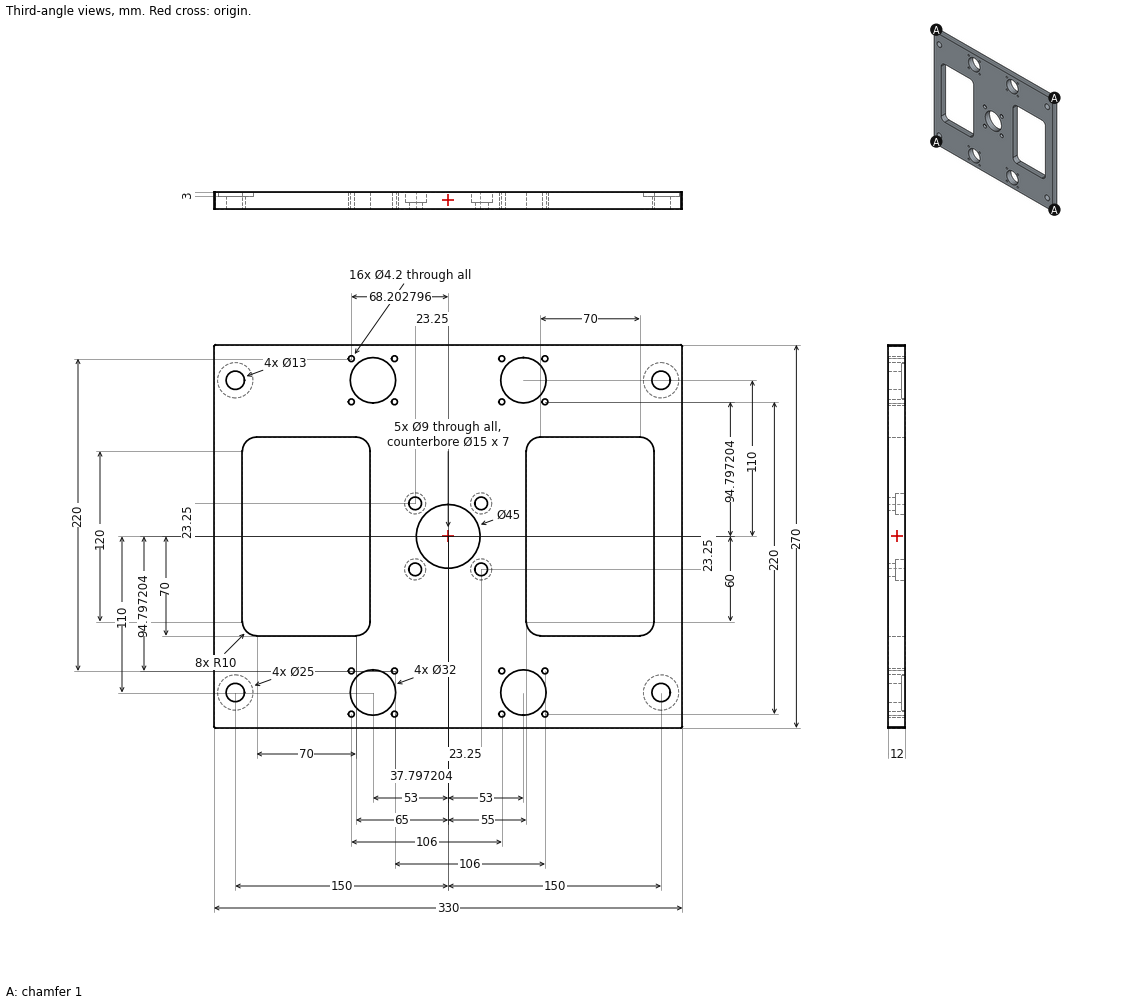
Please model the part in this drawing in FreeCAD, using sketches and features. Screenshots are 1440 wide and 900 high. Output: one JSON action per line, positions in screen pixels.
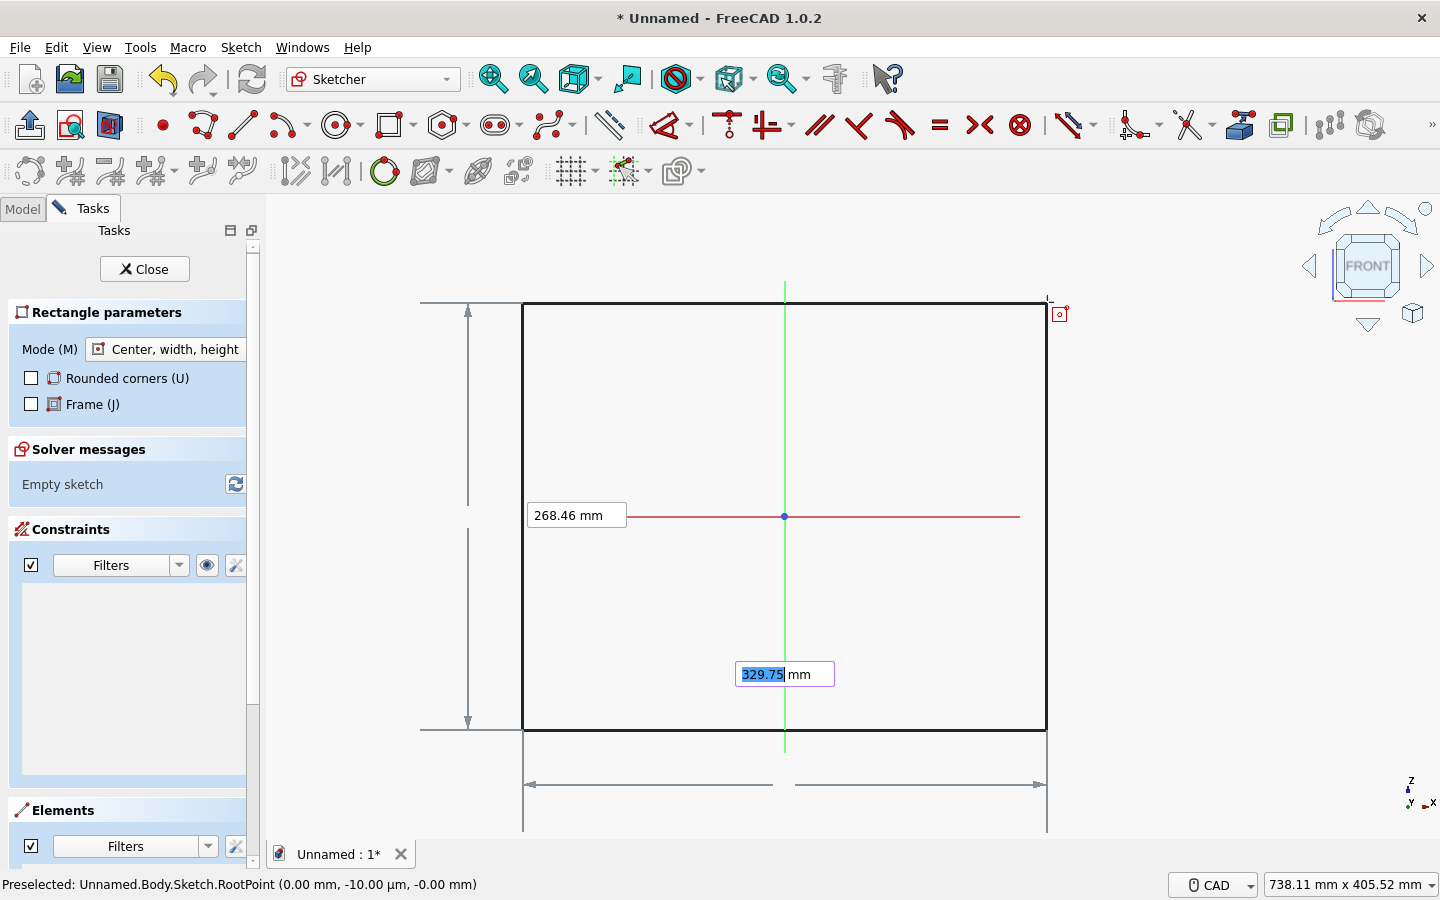
{"action": "type", "text": "330"}
{"action": "key", "text": "Tab"}
{"action": "type", "text": "270"}
{"action": "key", "text": "Return"}
{"action": "key", "text": "Escape"}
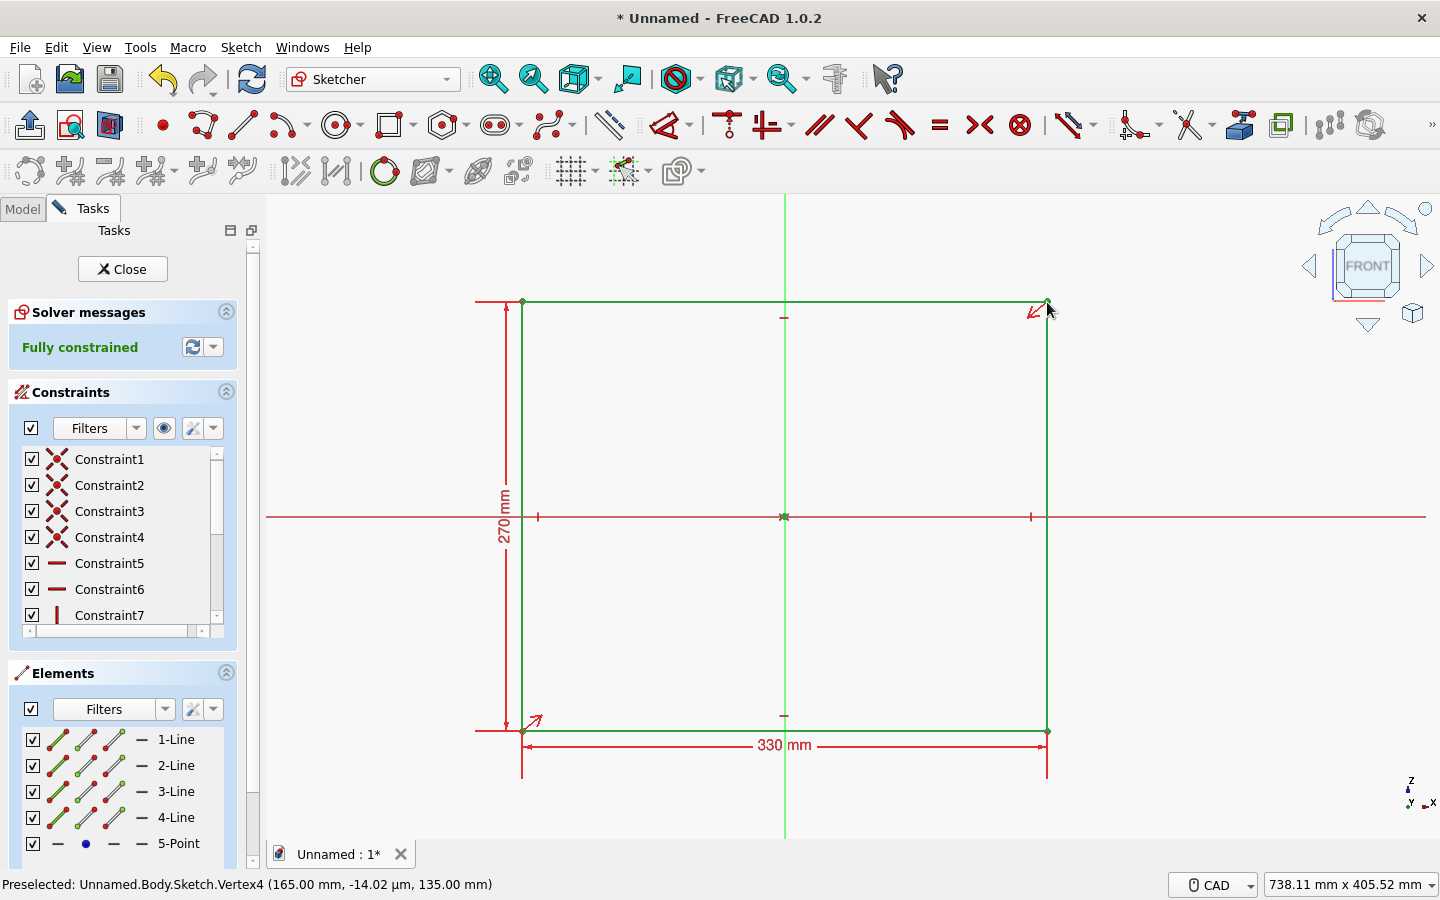
{"action": "left_click", "coordinate": [123, 269]}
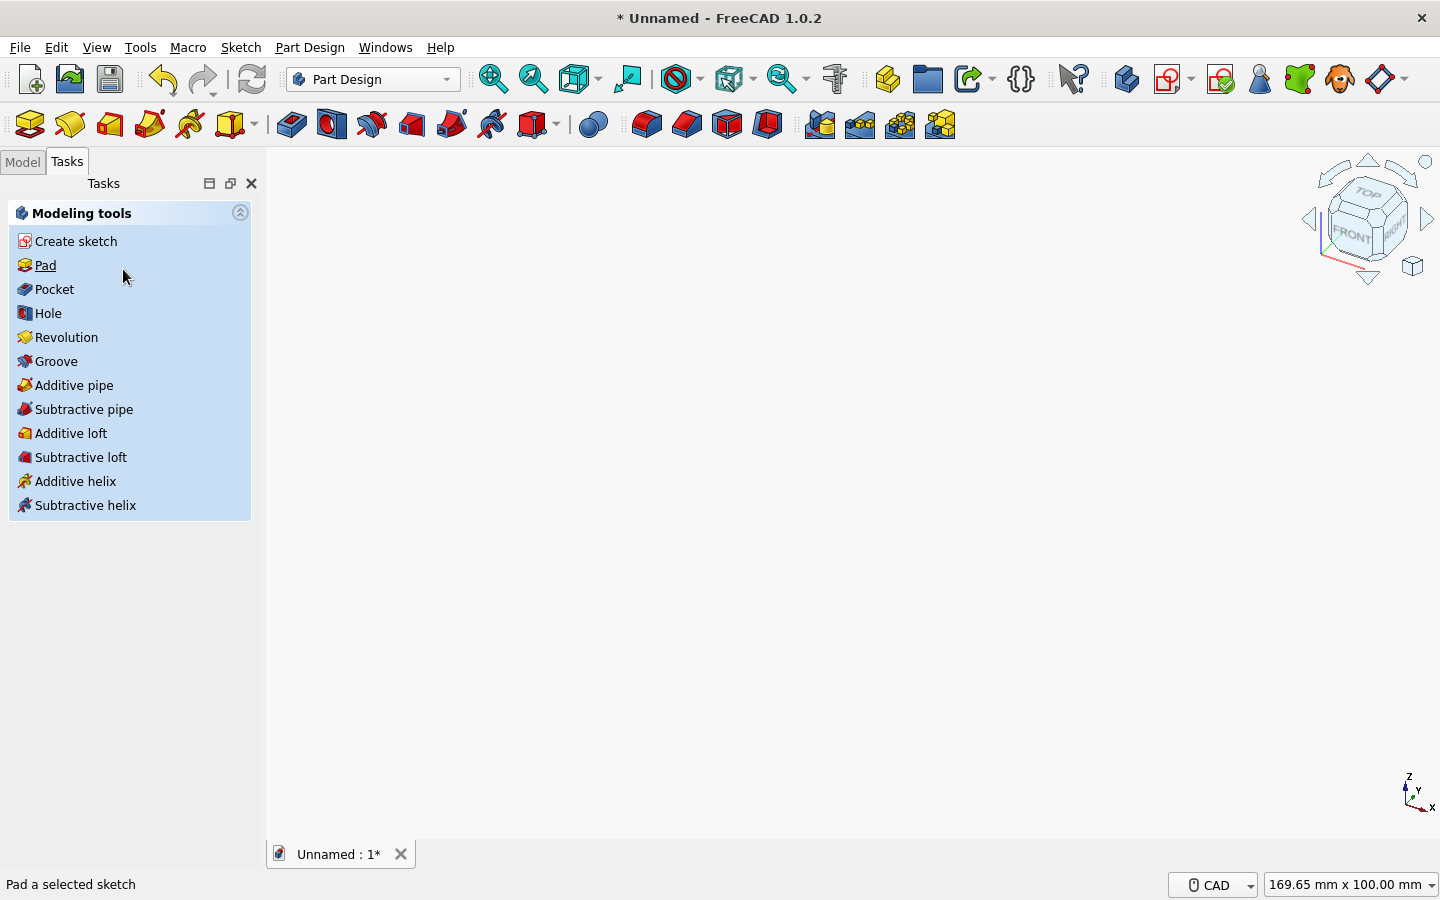
{"action": "left_click", "coordinate": [30, 124]}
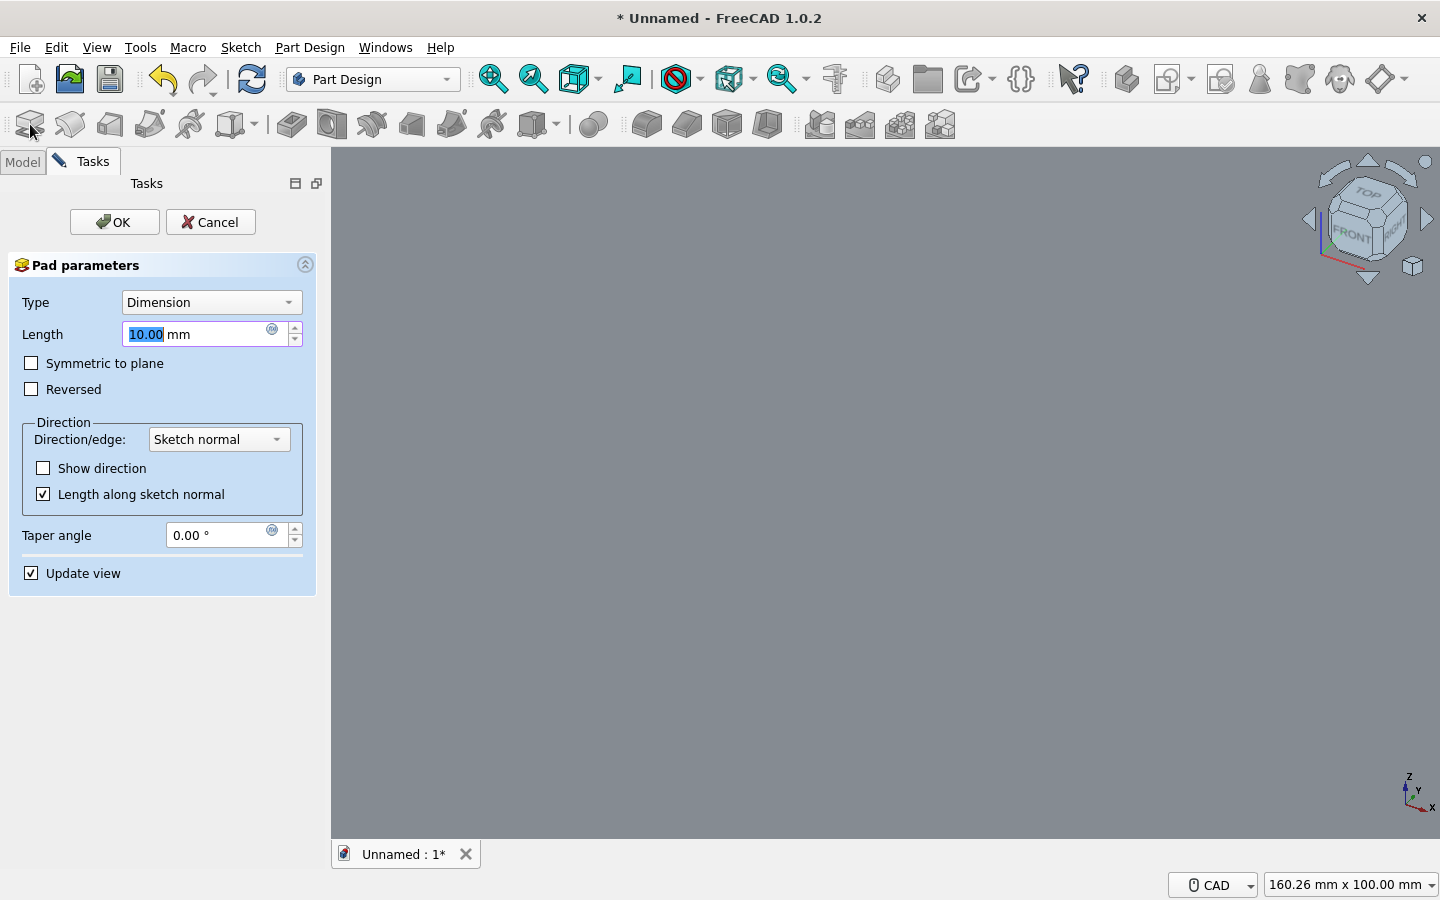
{"action": "type", "text": "12"}
{"action": "key", "text": "Tab"}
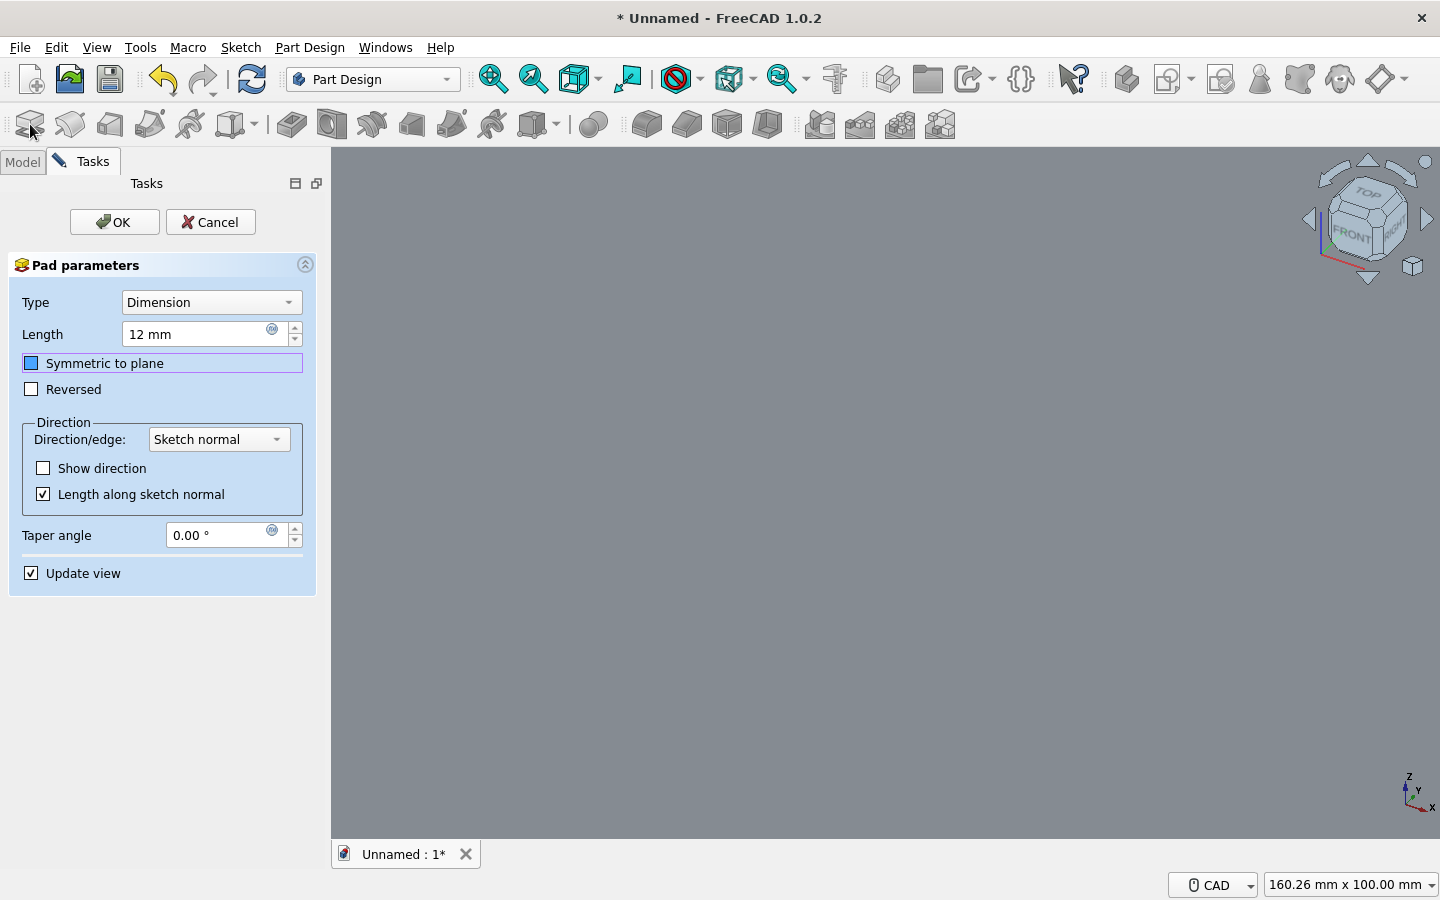
{"action": "left_click", "coordinate": [30, 363]}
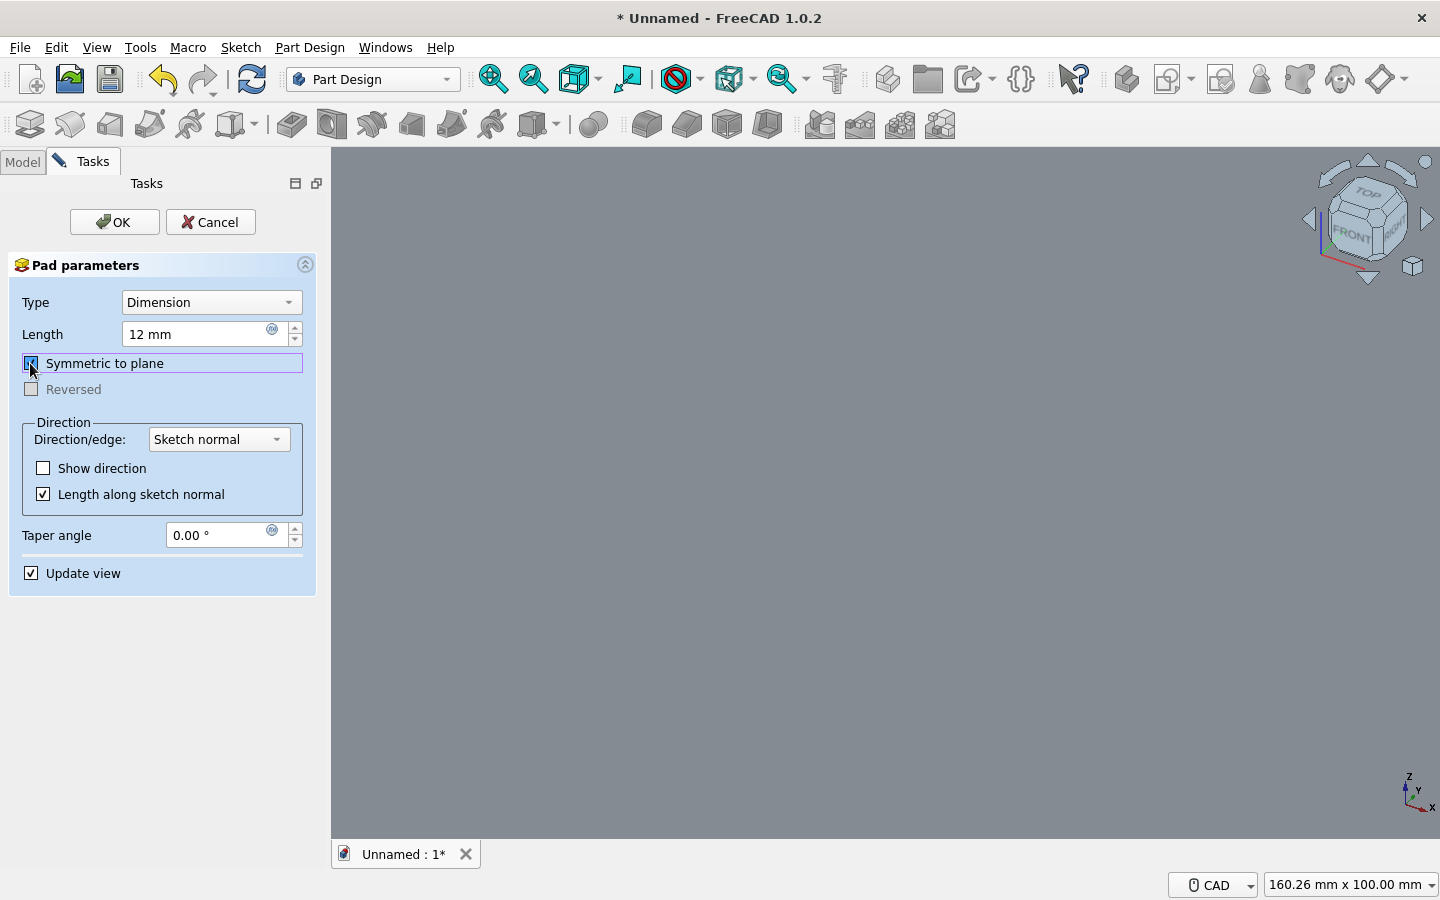
{"action": "left_click", "coordinate": [115, 222]}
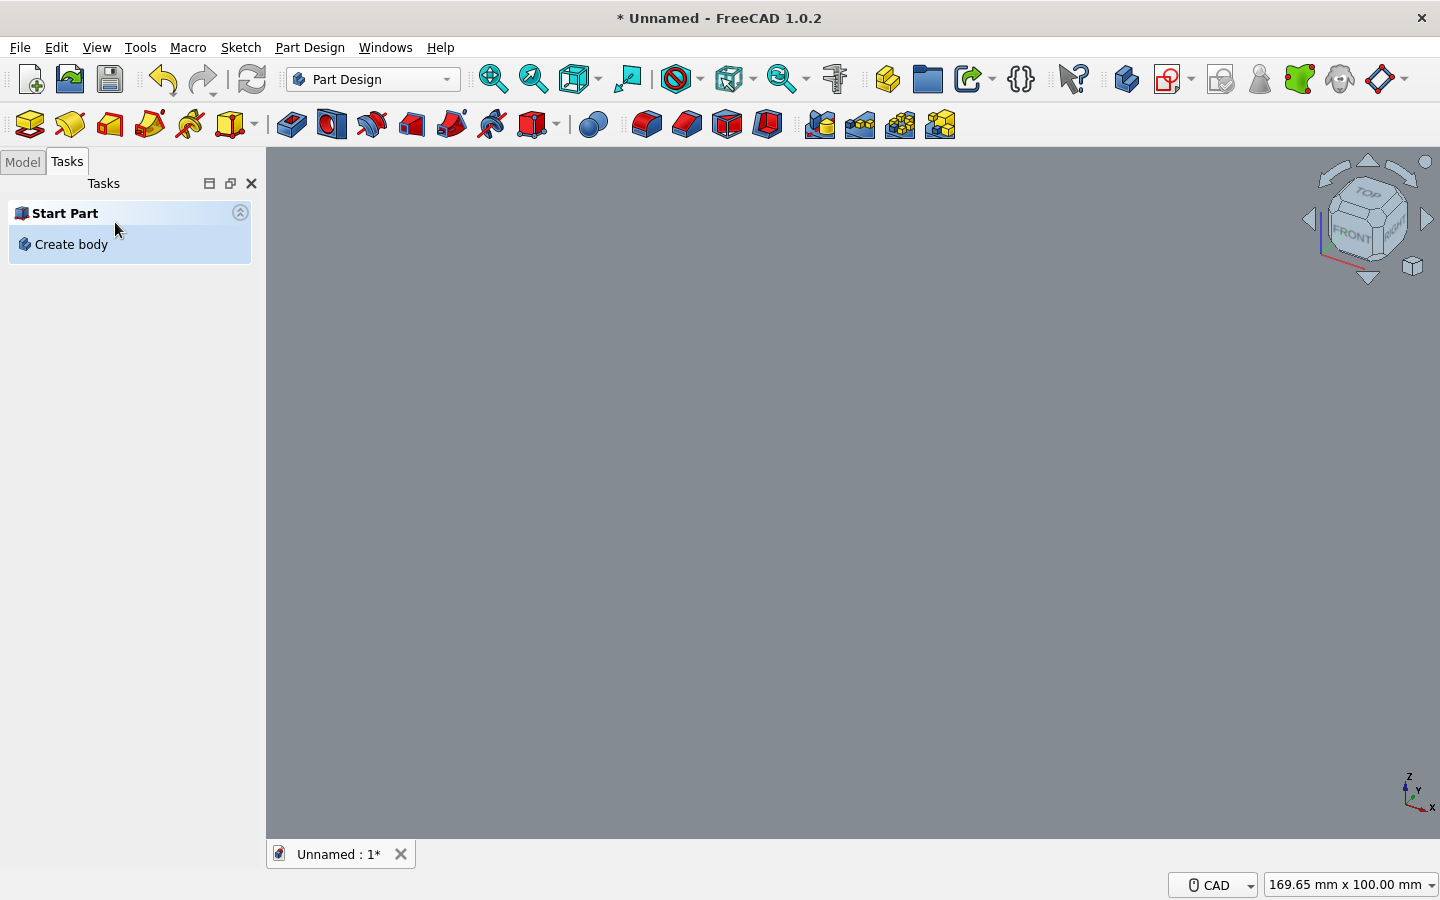
{"action": "left_click", "coordinate": [494, 80]}